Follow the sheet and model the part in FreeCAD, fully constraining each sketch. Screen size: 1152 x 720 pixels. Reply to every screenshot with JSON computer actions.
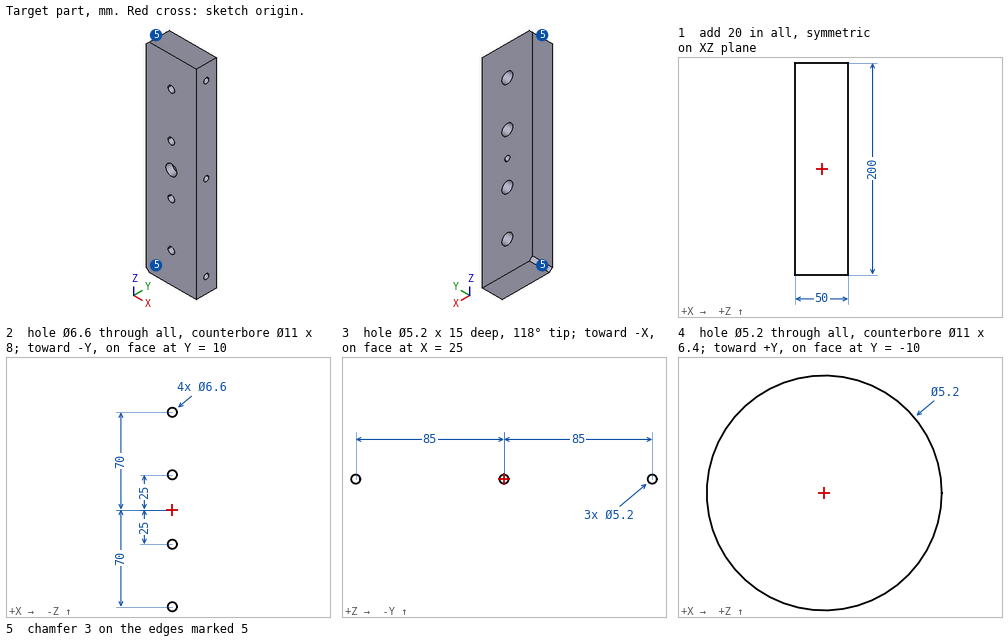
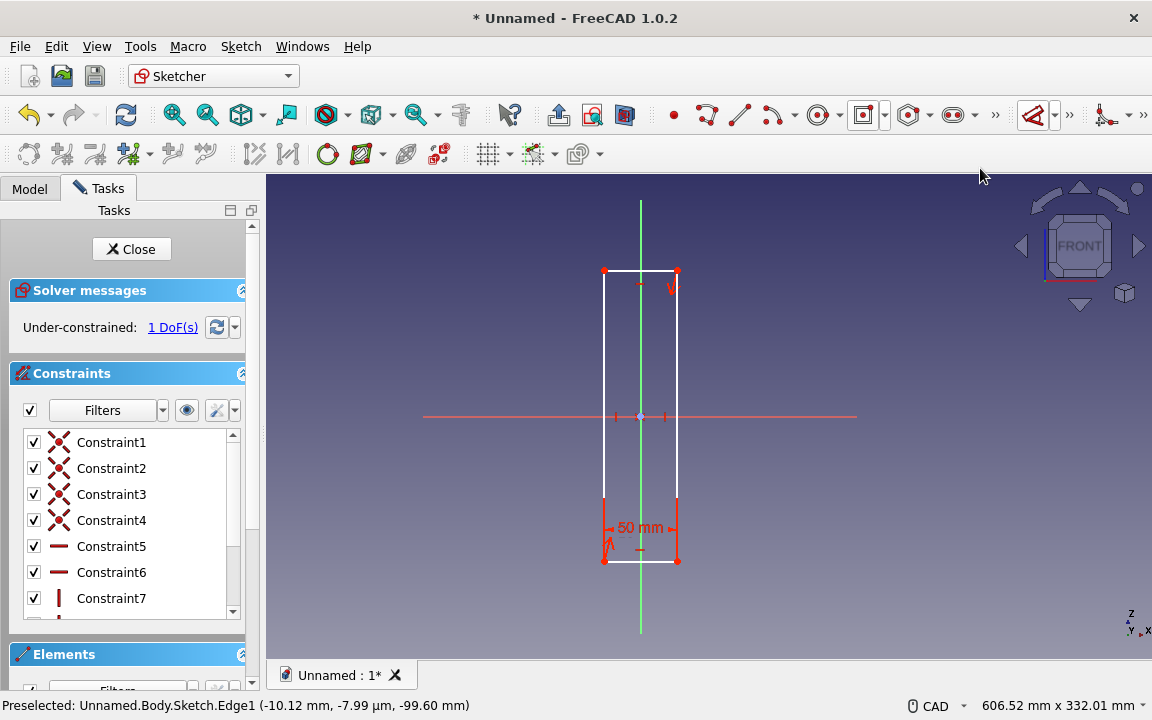
{"action": "left_click", "coordinate": [677, 475]}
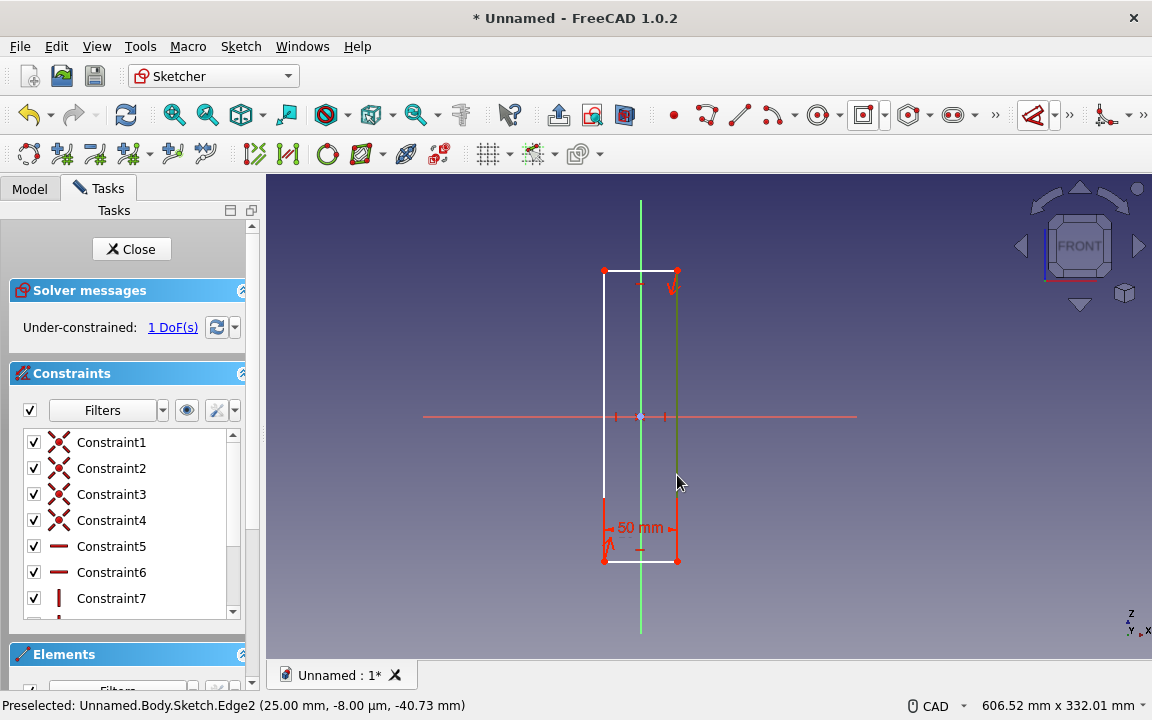
{"action": "key", "text": "i"}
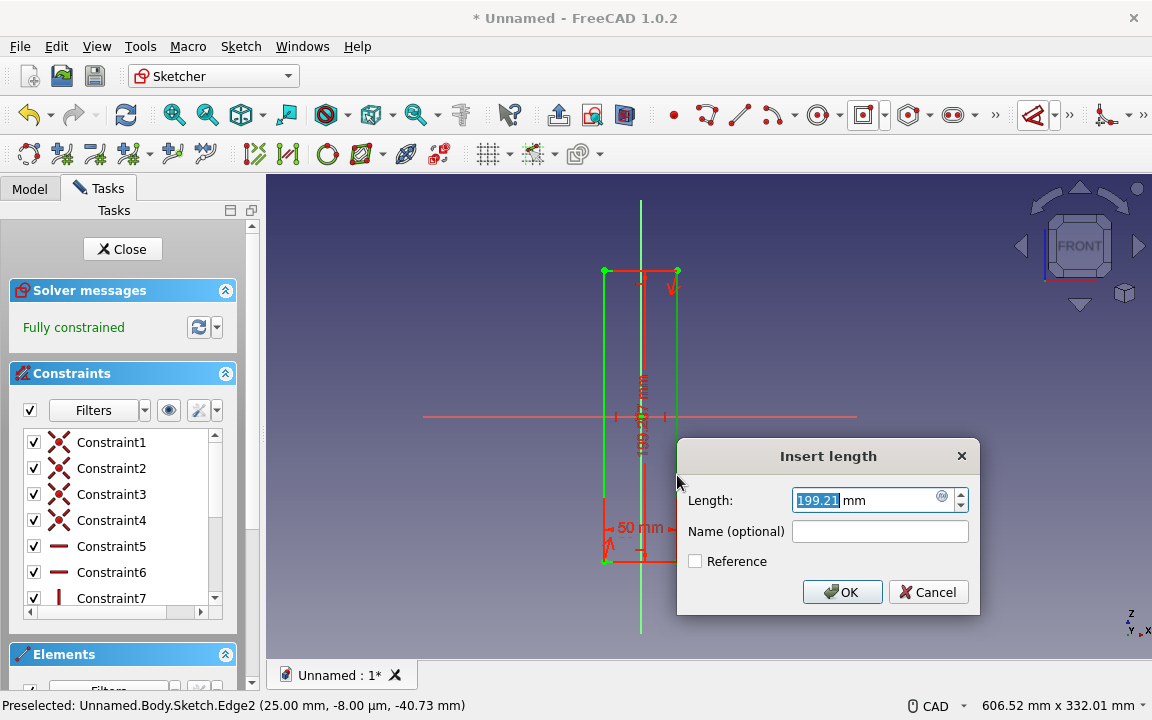
{"action": "type", "text": "200"}
{"action": "key", "text": "Return"}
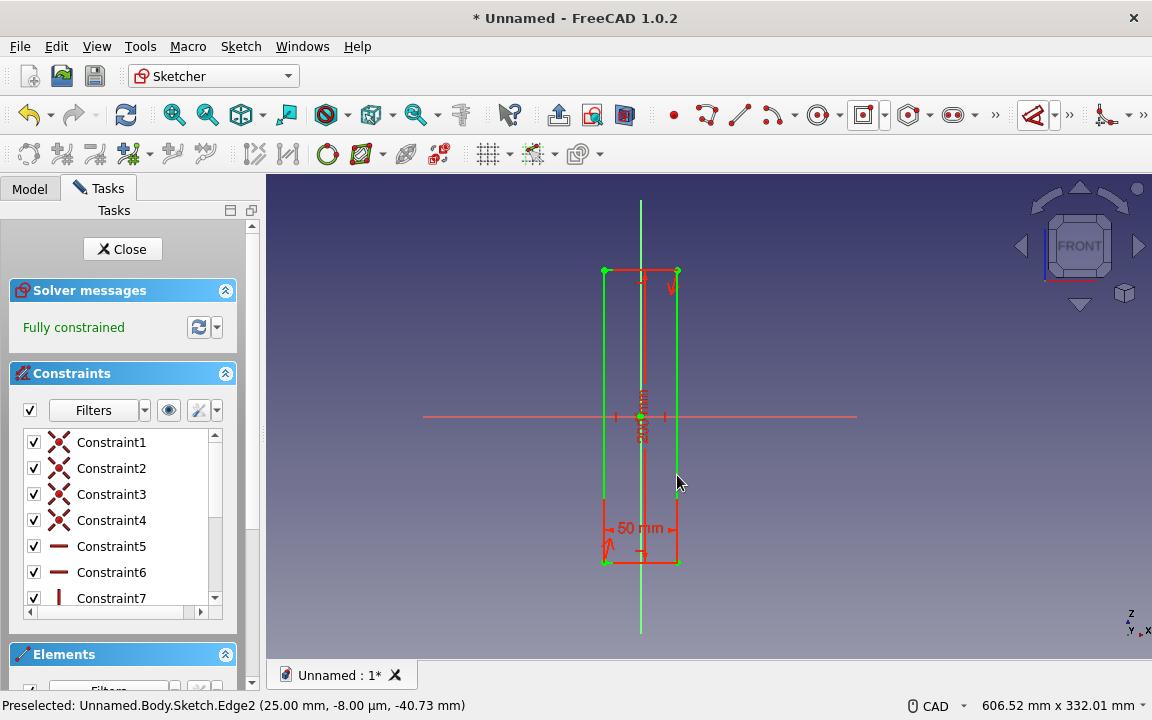
{"action": "left_click", "coordinate": [123, 249]}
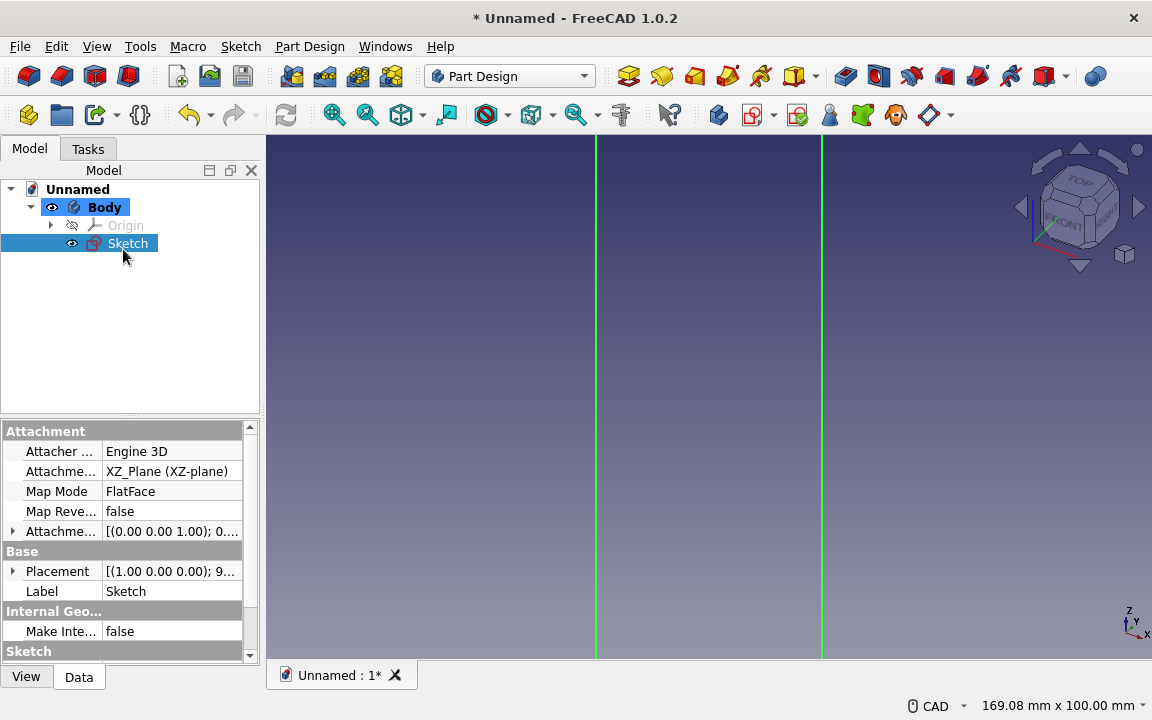
{"action": "left_click", "coordinate": [629, 76]}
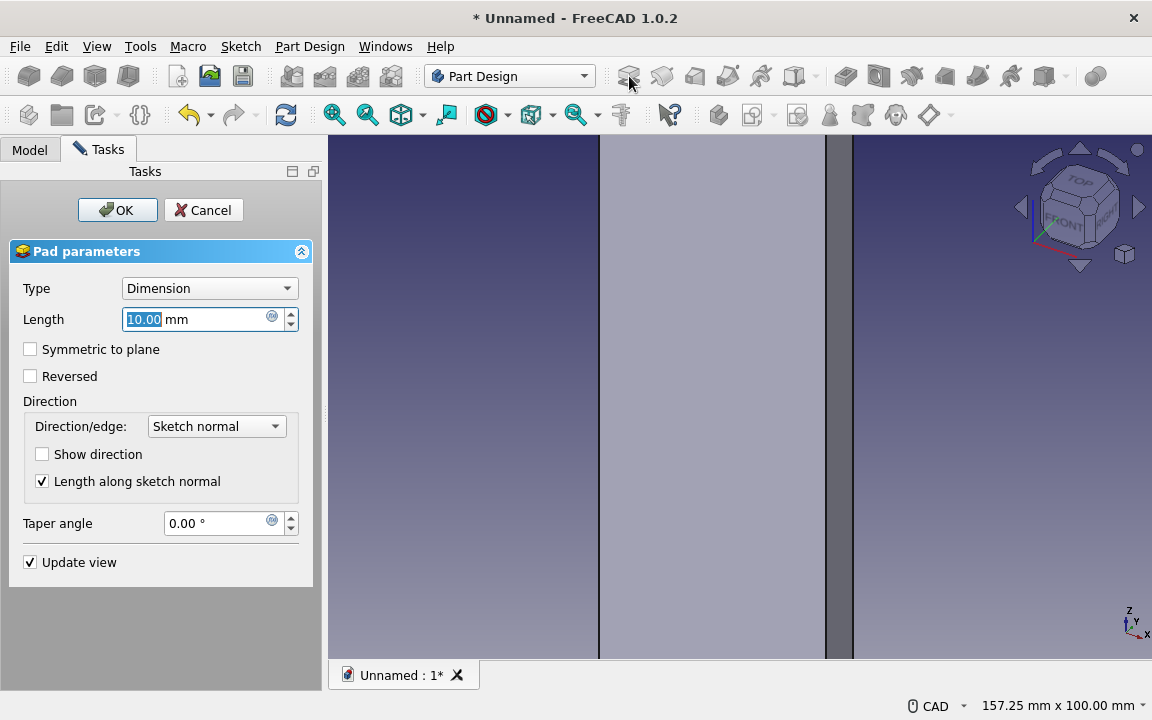
{"action": "type", "text": "20"}
{"action": "key", "text": "Tab"}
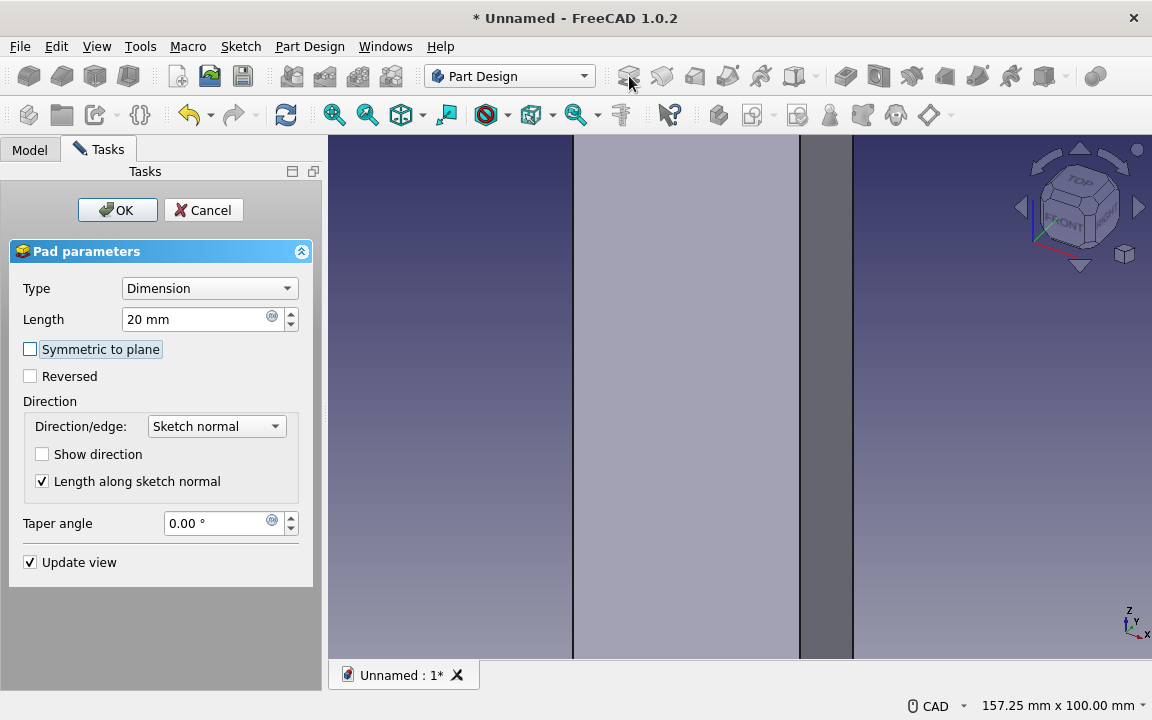
{"action": "left_click", "coordinate": [31, 349]}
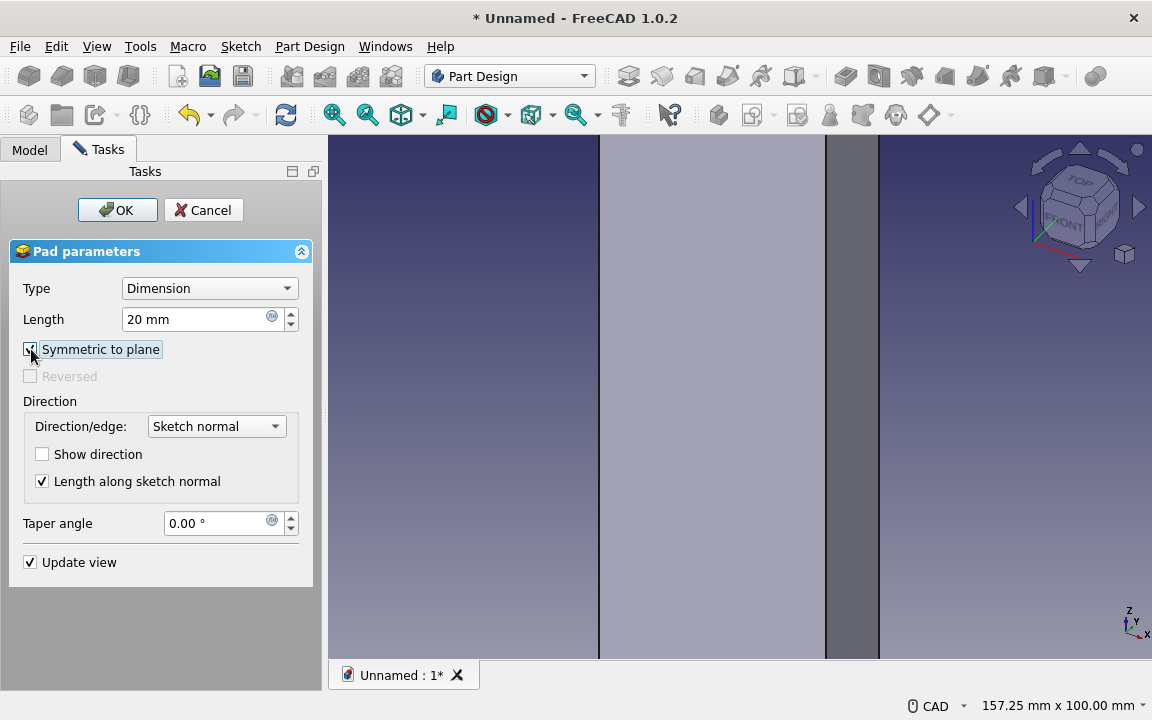
{"action": "left_click", "coordinate": [118, 210]}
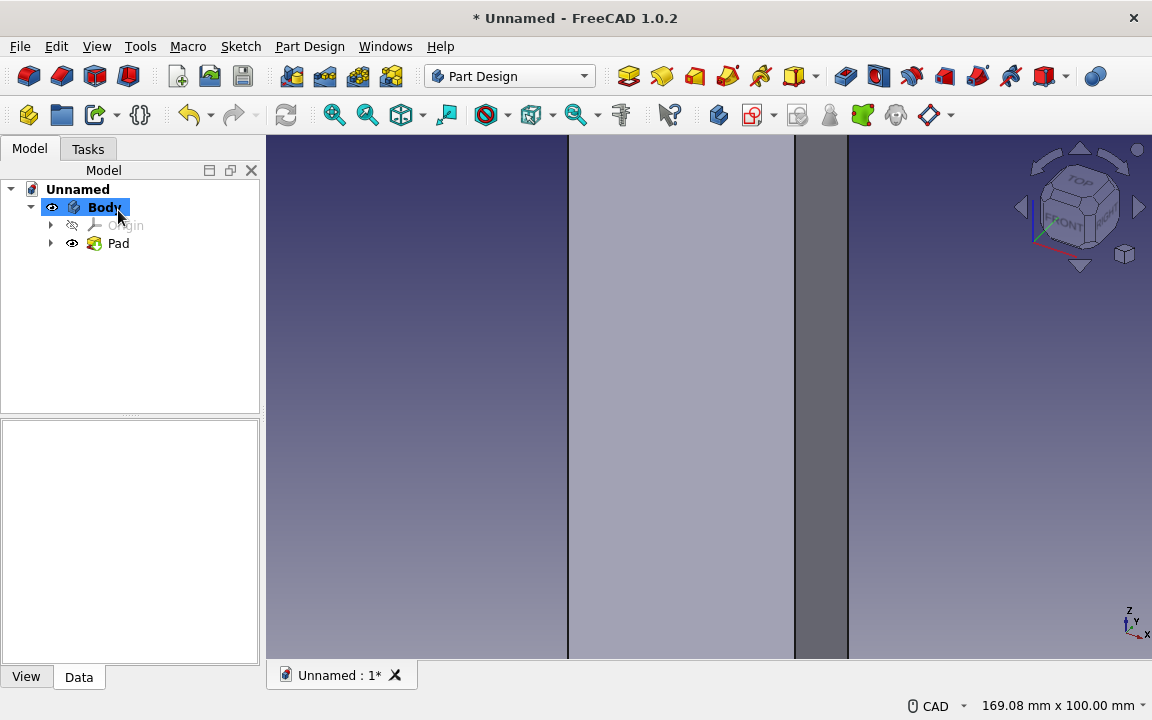
{"action": "left_click", "coordinate": [335, 116]}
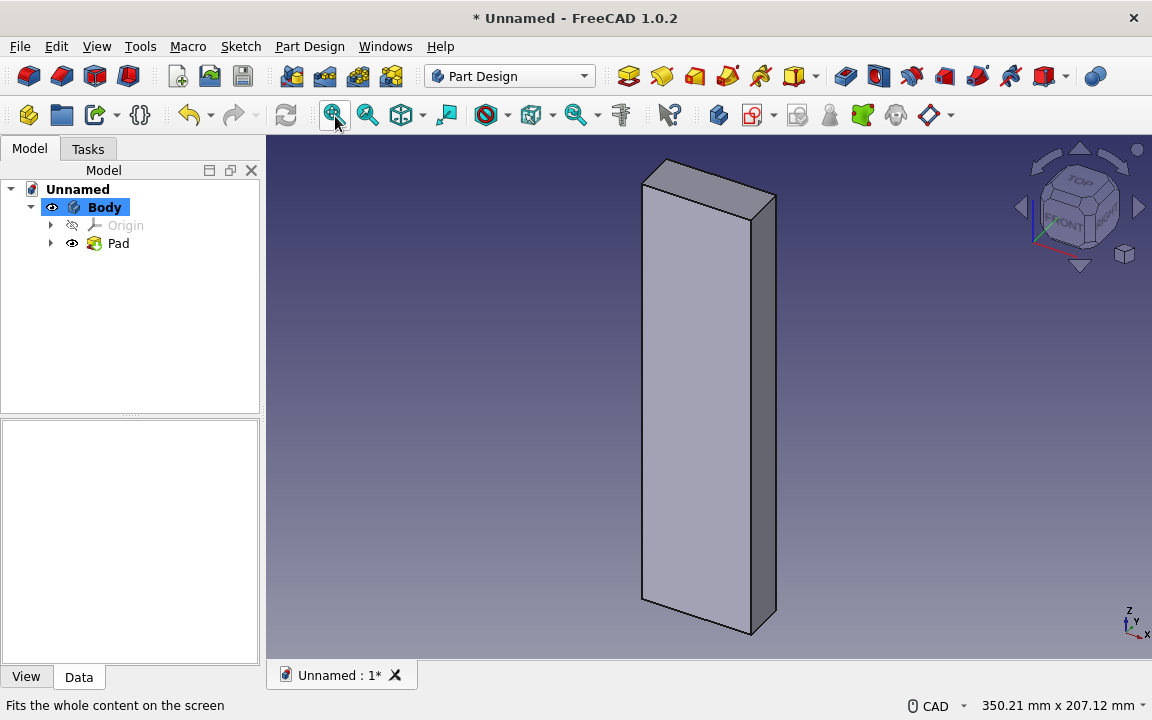
{"action": "key", "text": "4"}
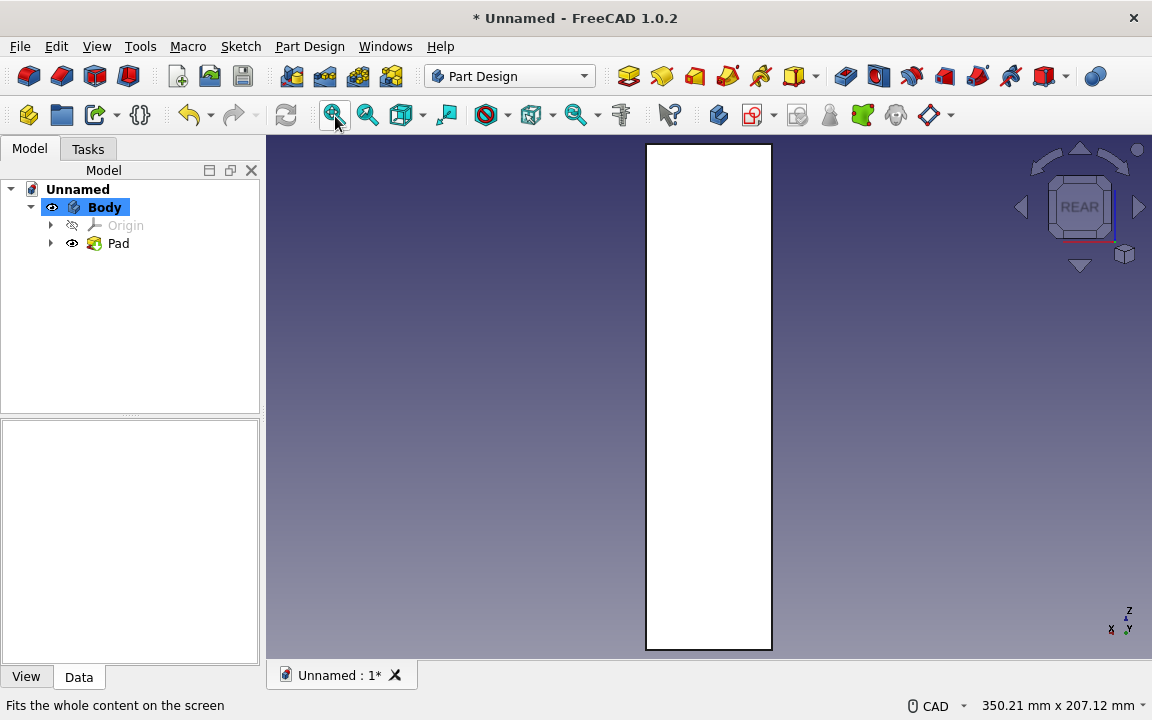
{"action": "left_click", "coordinate": [709, 251]}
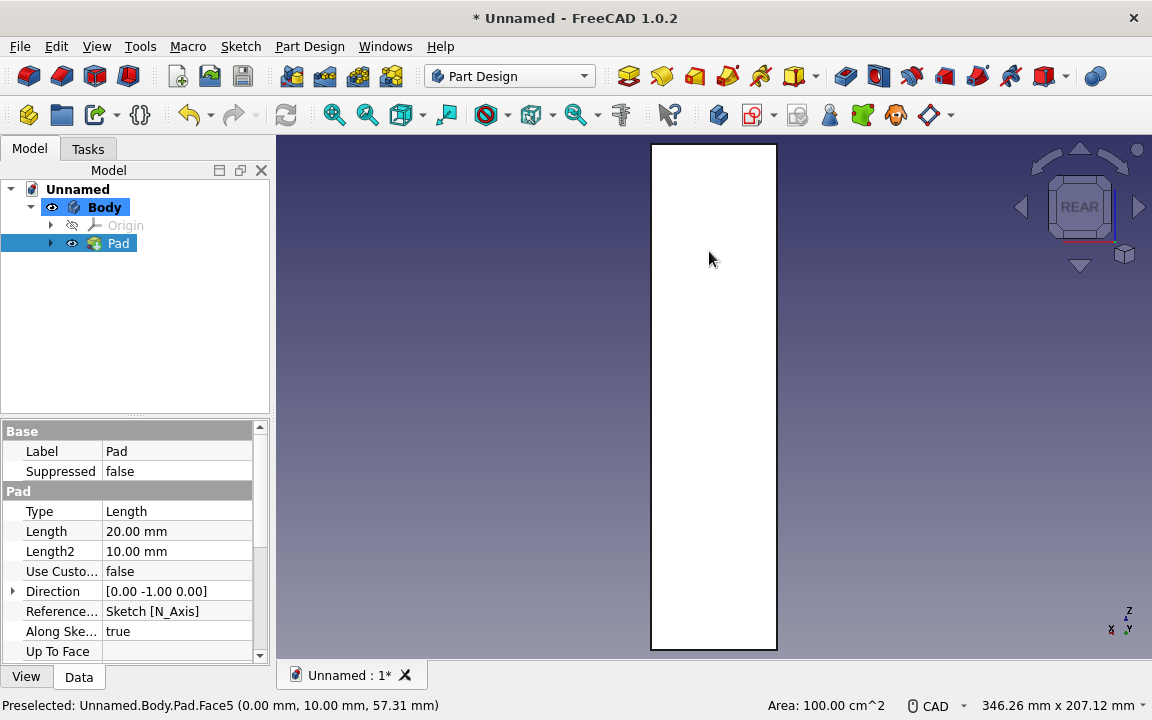
{"action": "left_click", "coordinate": [752, 116]}